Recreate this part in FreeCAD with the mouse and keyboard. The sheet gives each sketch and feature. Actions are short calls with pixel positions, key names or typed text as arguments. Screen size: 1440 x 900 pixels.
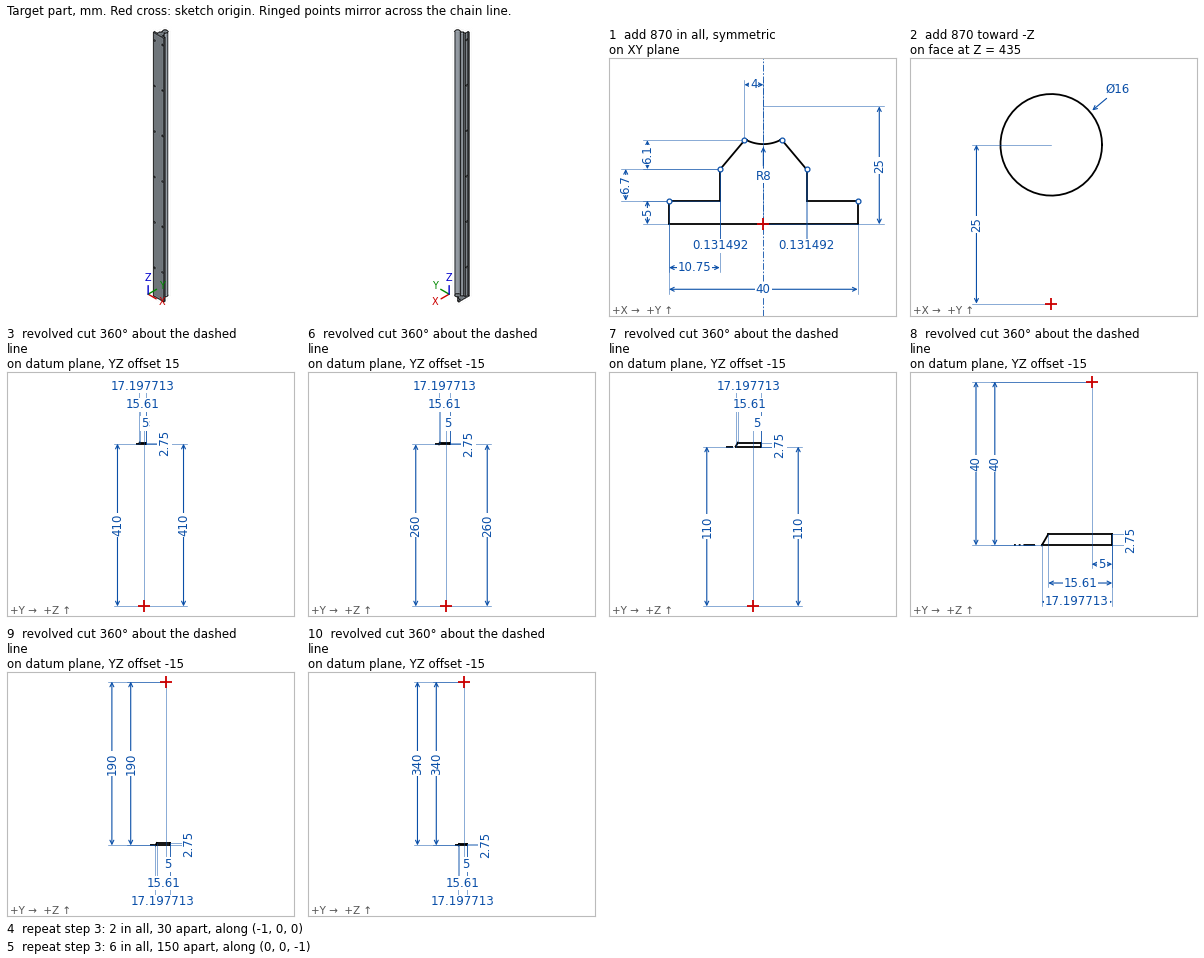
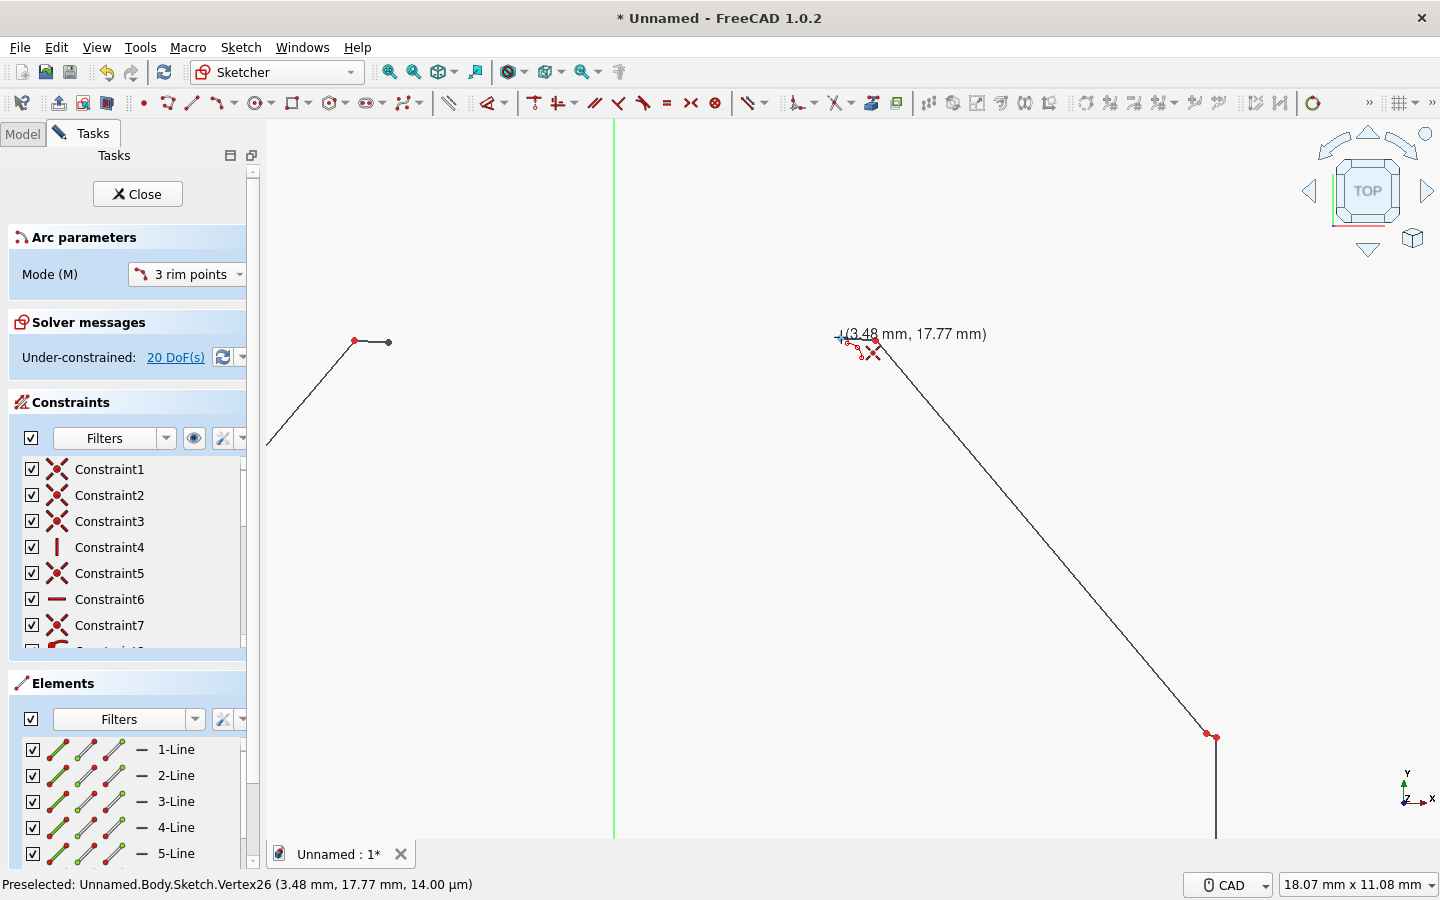
click(841, 339)
click(388, 342)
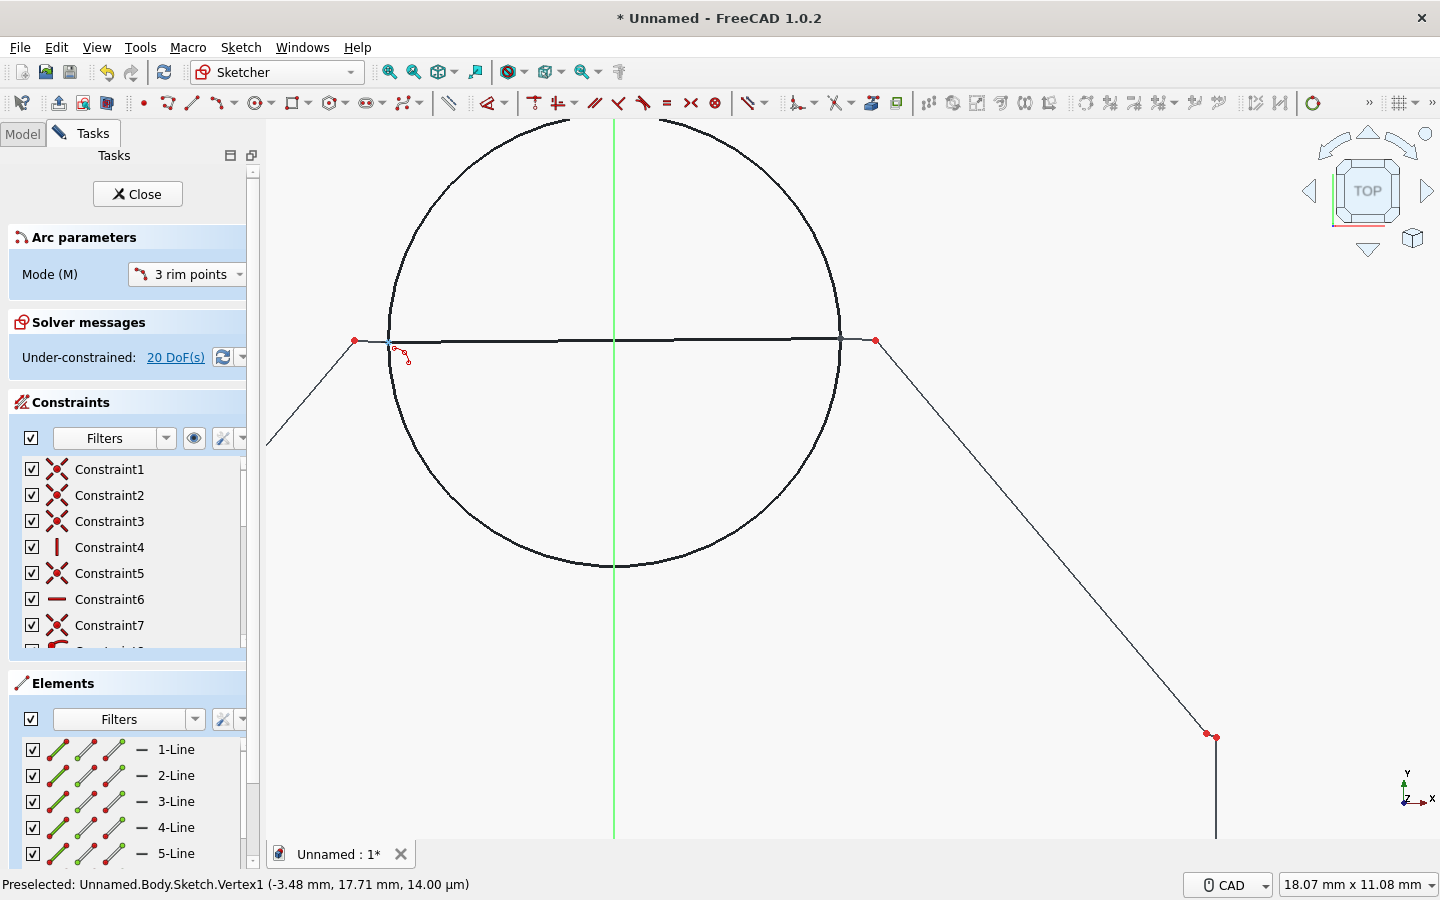
scroll(840, 336, down, 7)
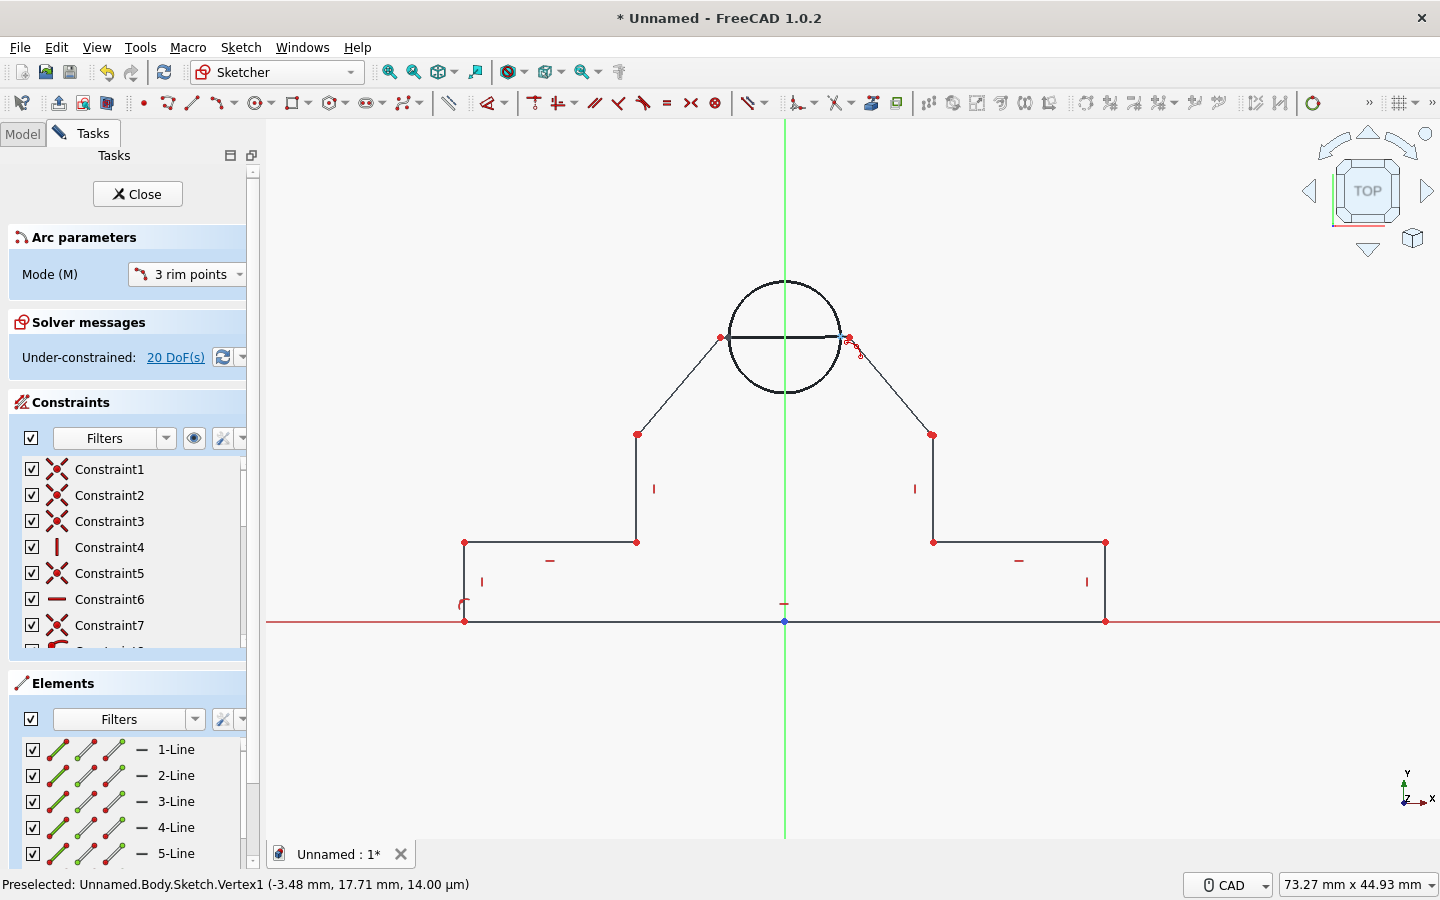
scroll(773, 349, up, 2)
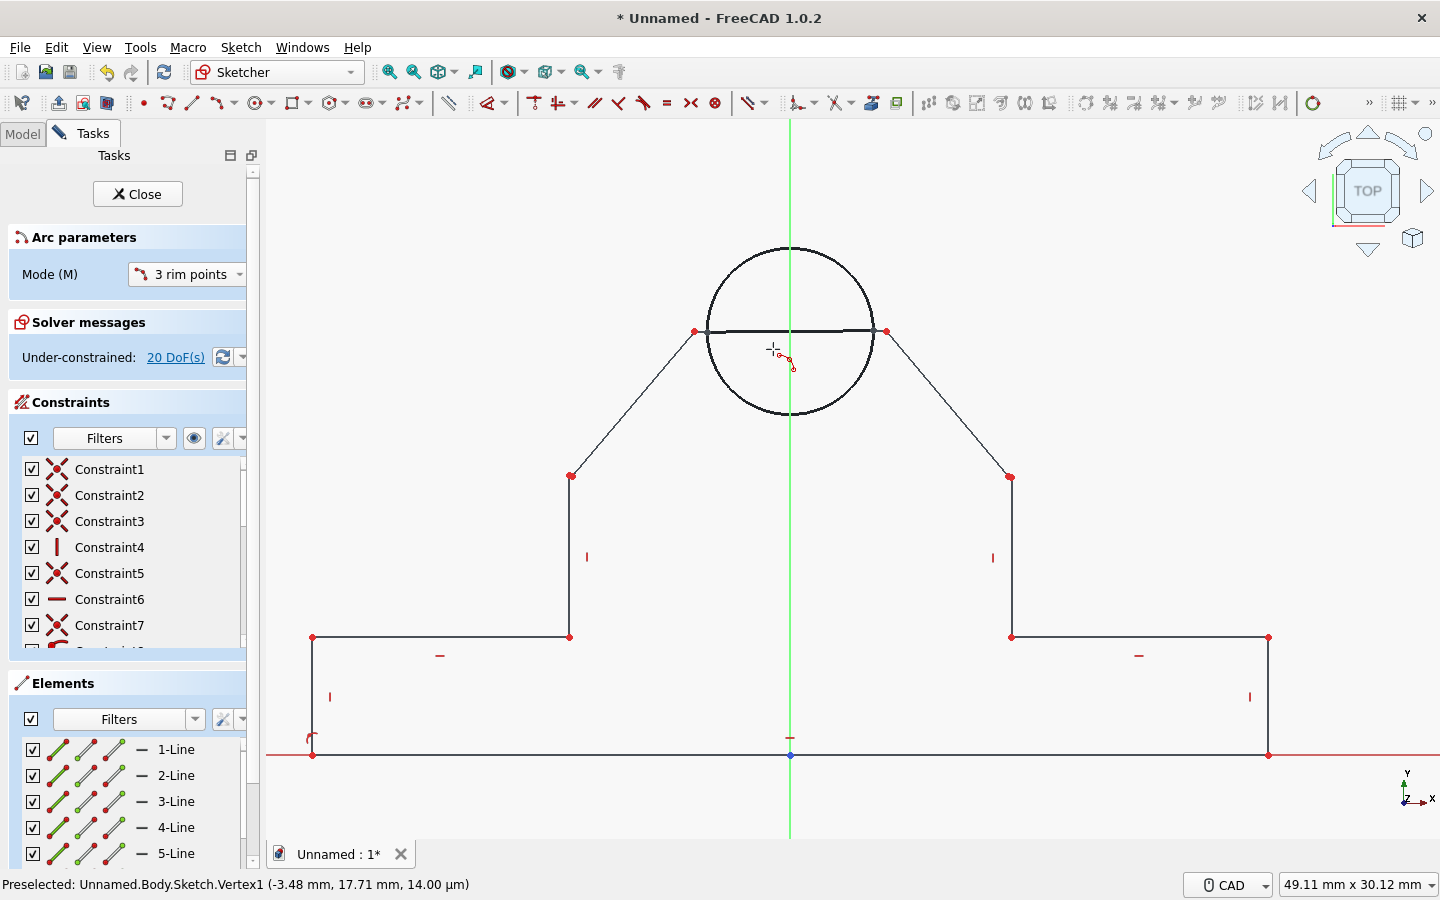
click(773, 348)
key(Escape)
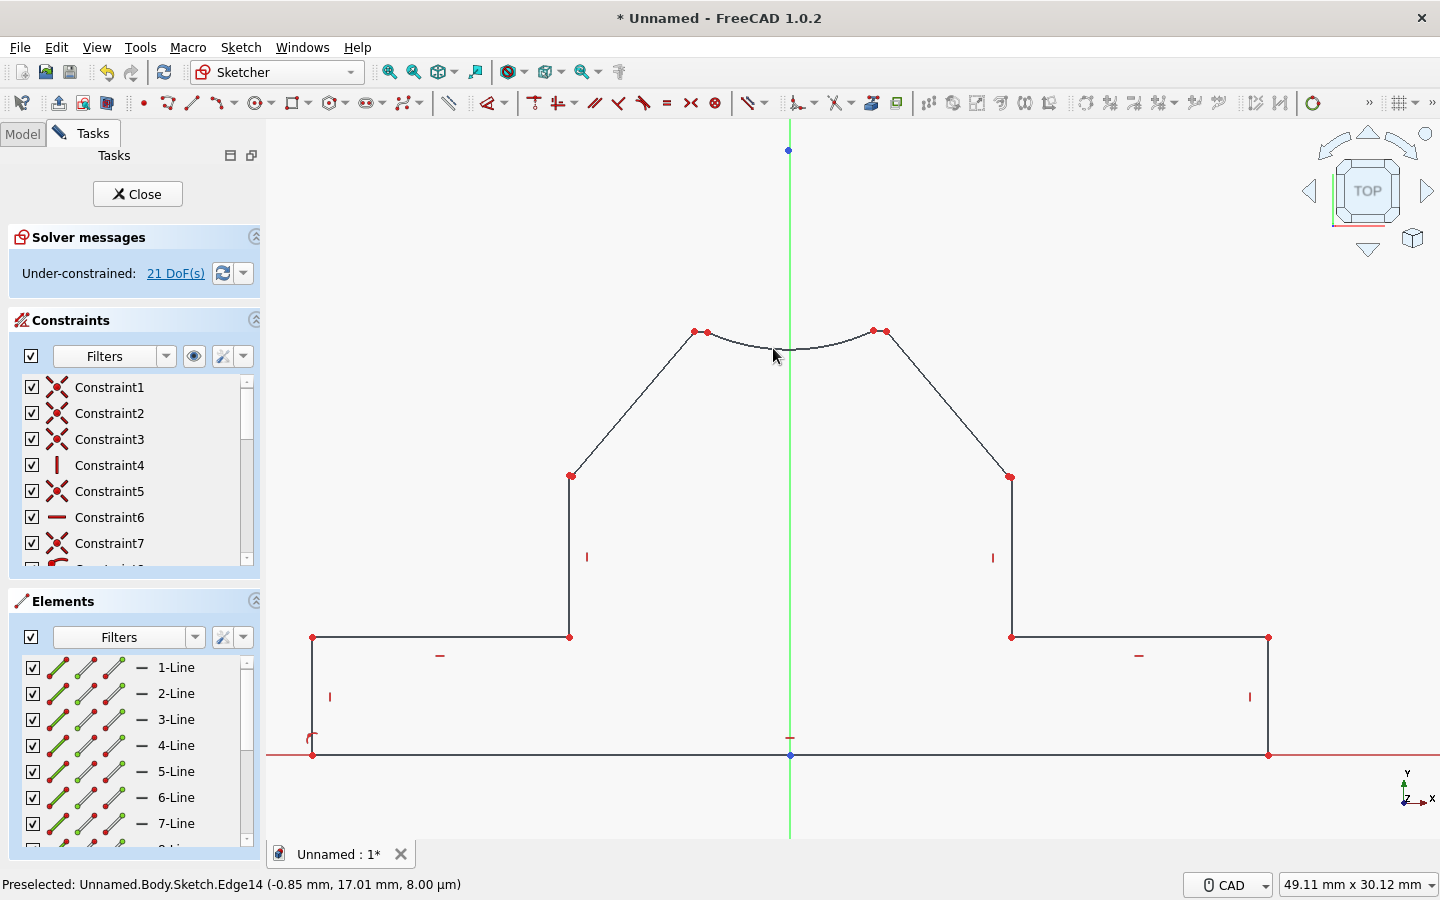
scroll(701, 332, up, 5)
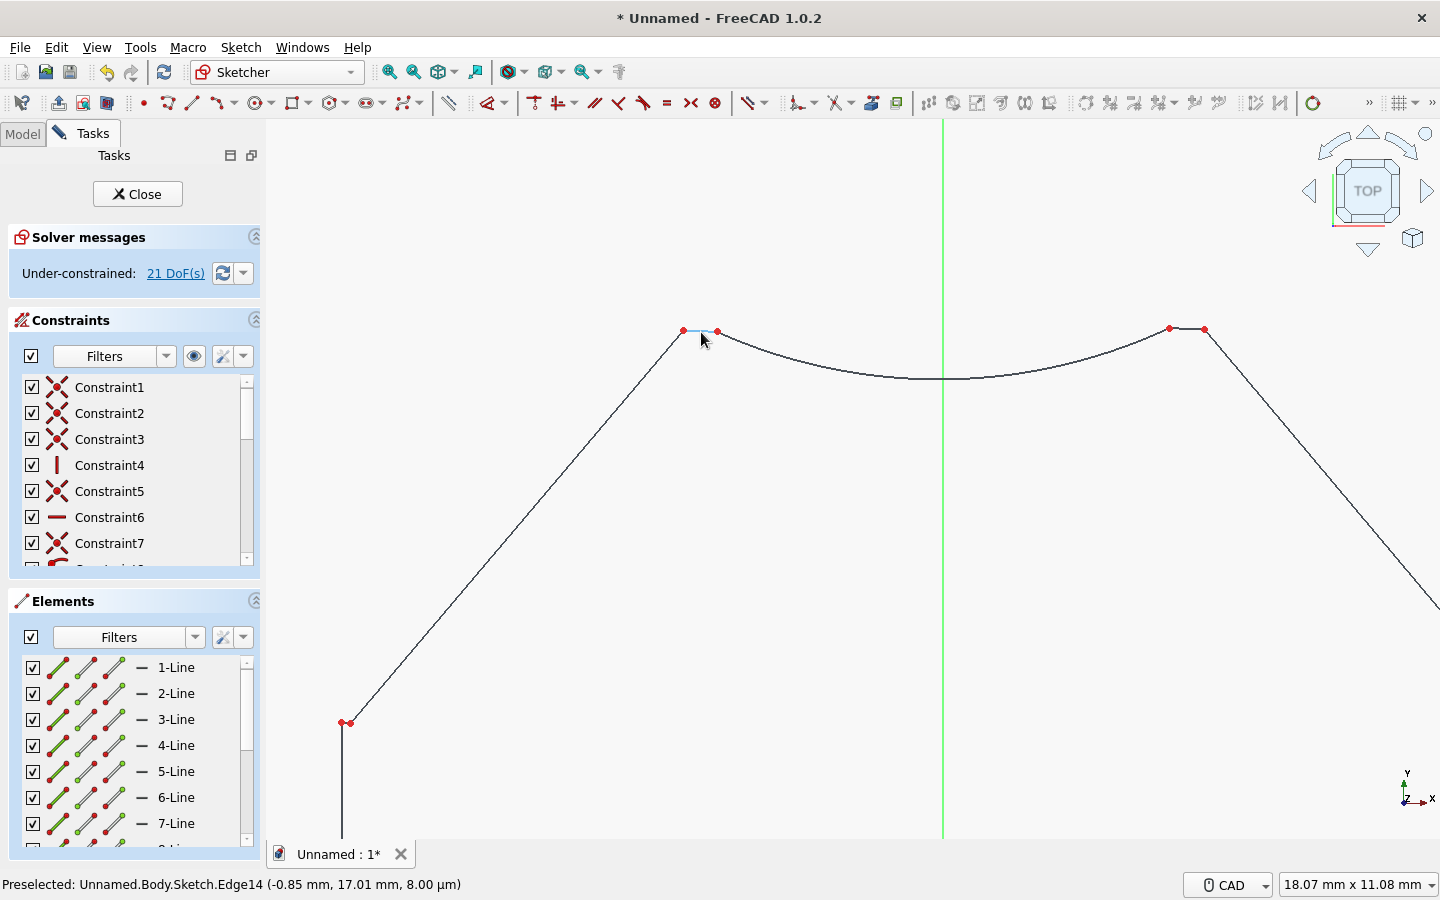
click(700, 331)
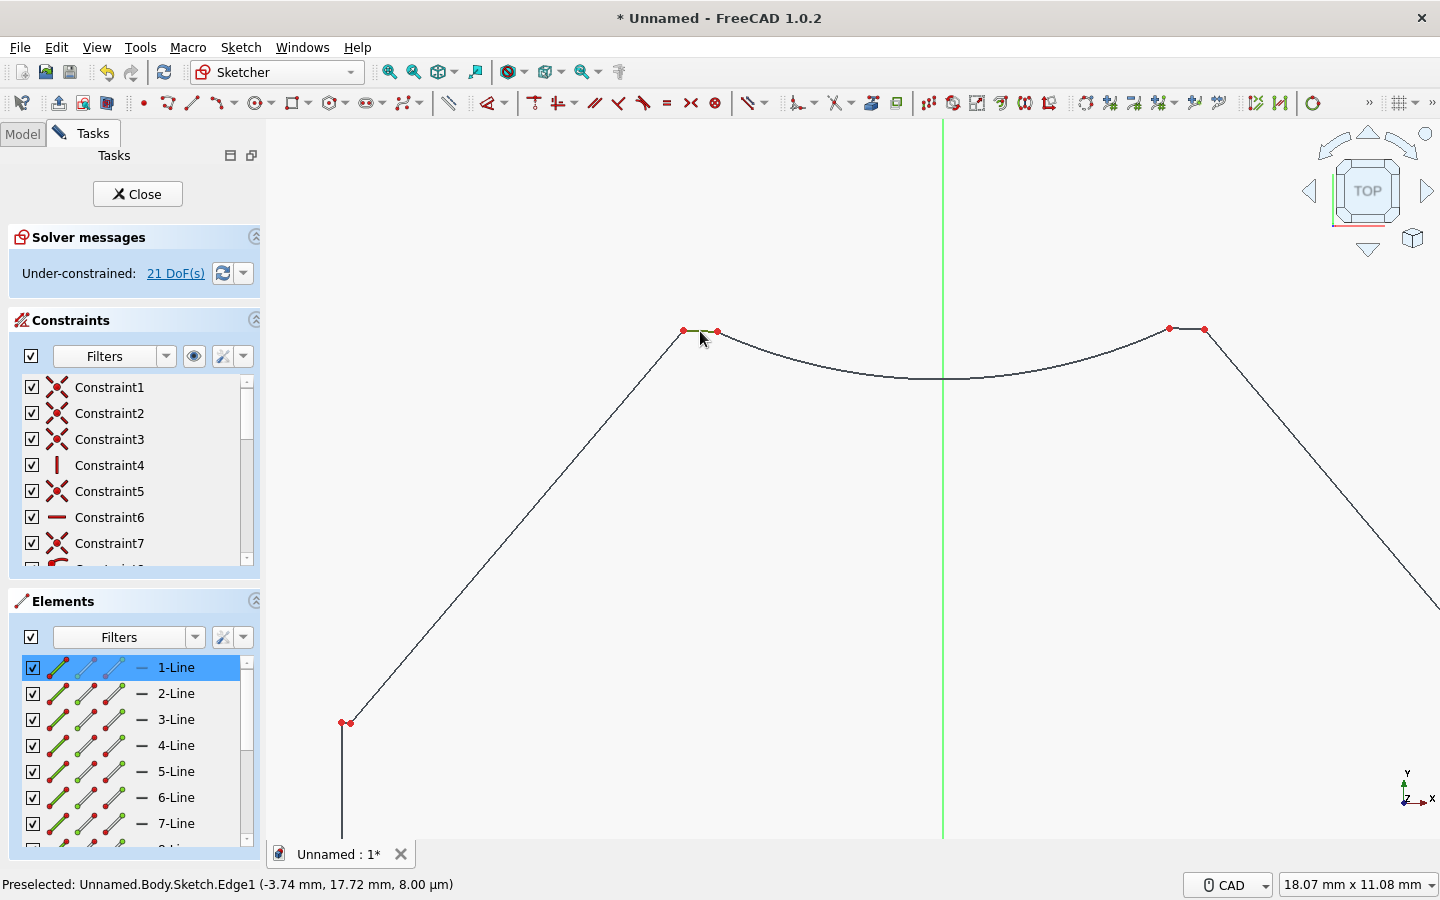
click(576, 104)